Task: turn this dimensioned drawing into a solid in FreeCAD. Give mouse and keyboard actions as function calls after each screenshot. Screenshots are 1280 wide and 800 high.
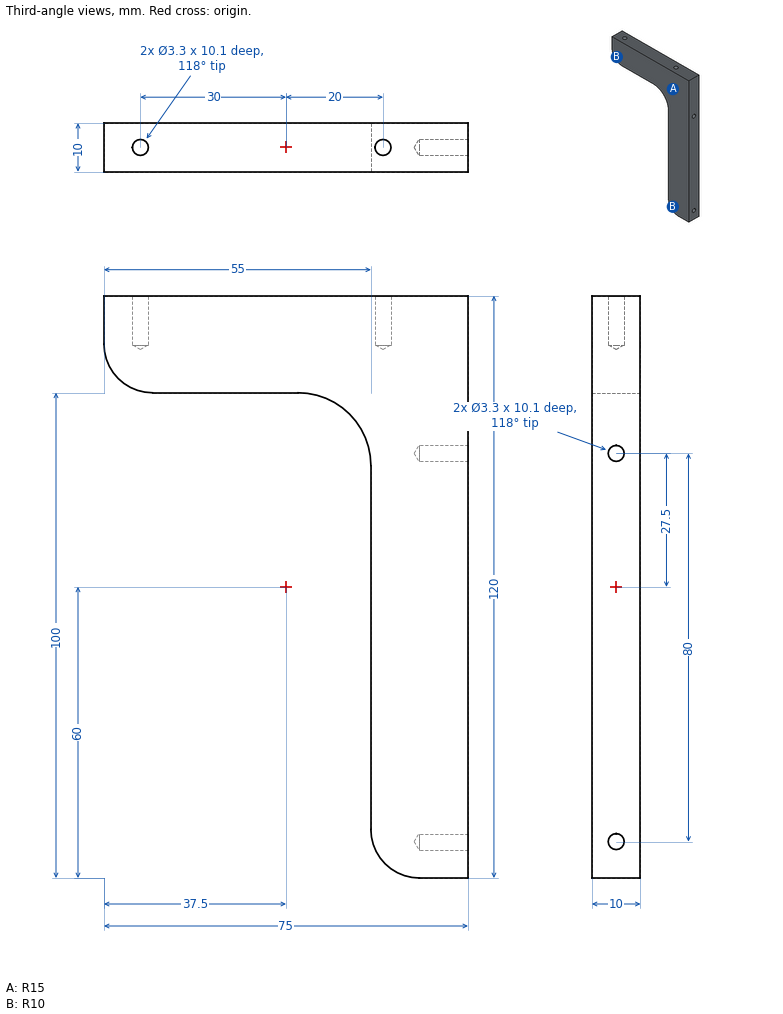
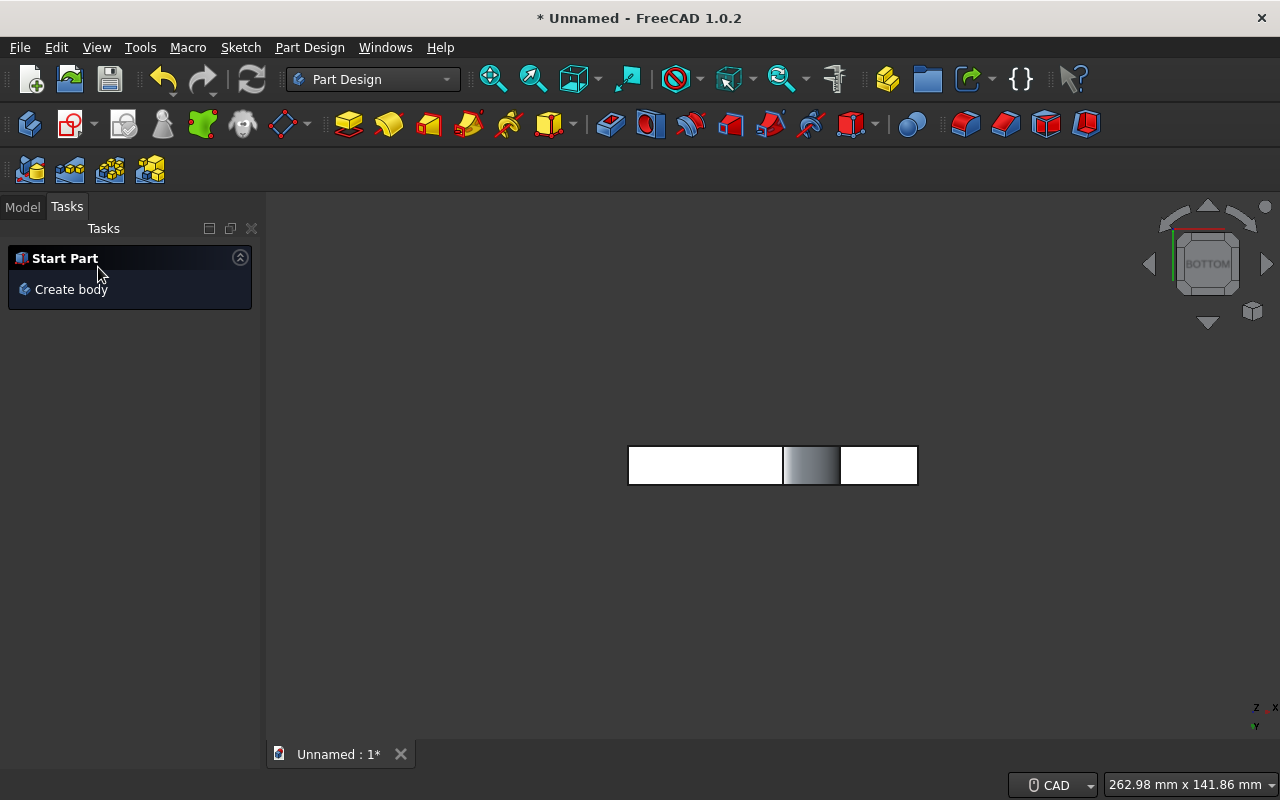
click(840, 464)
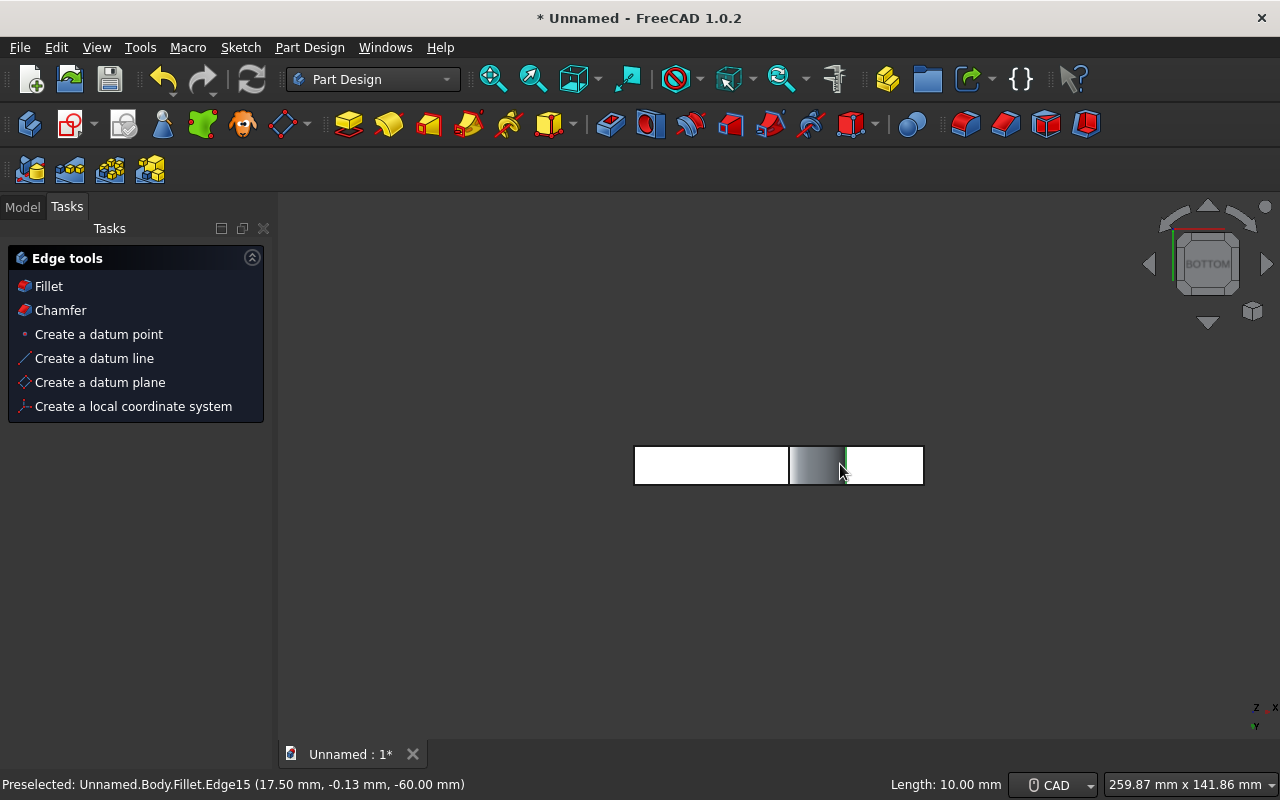
click(634, 464, ctrl)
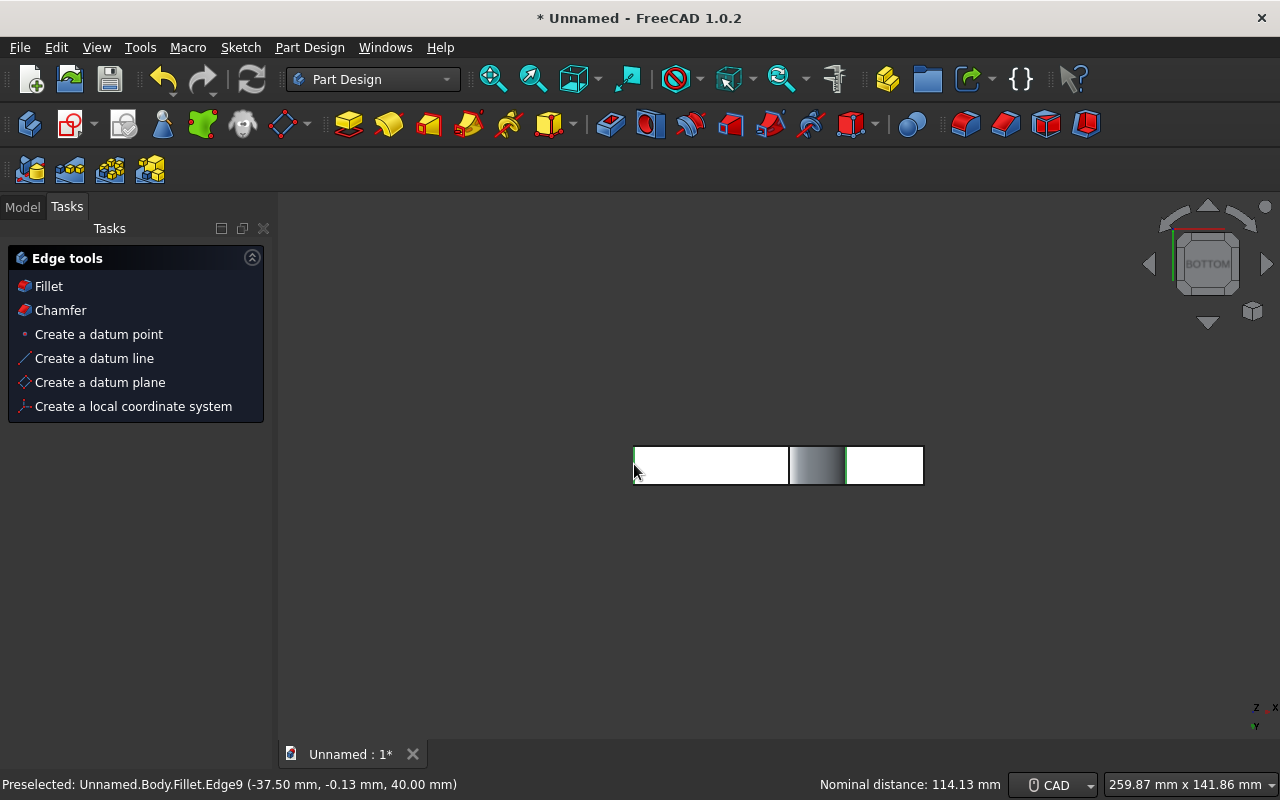
click(966, 124)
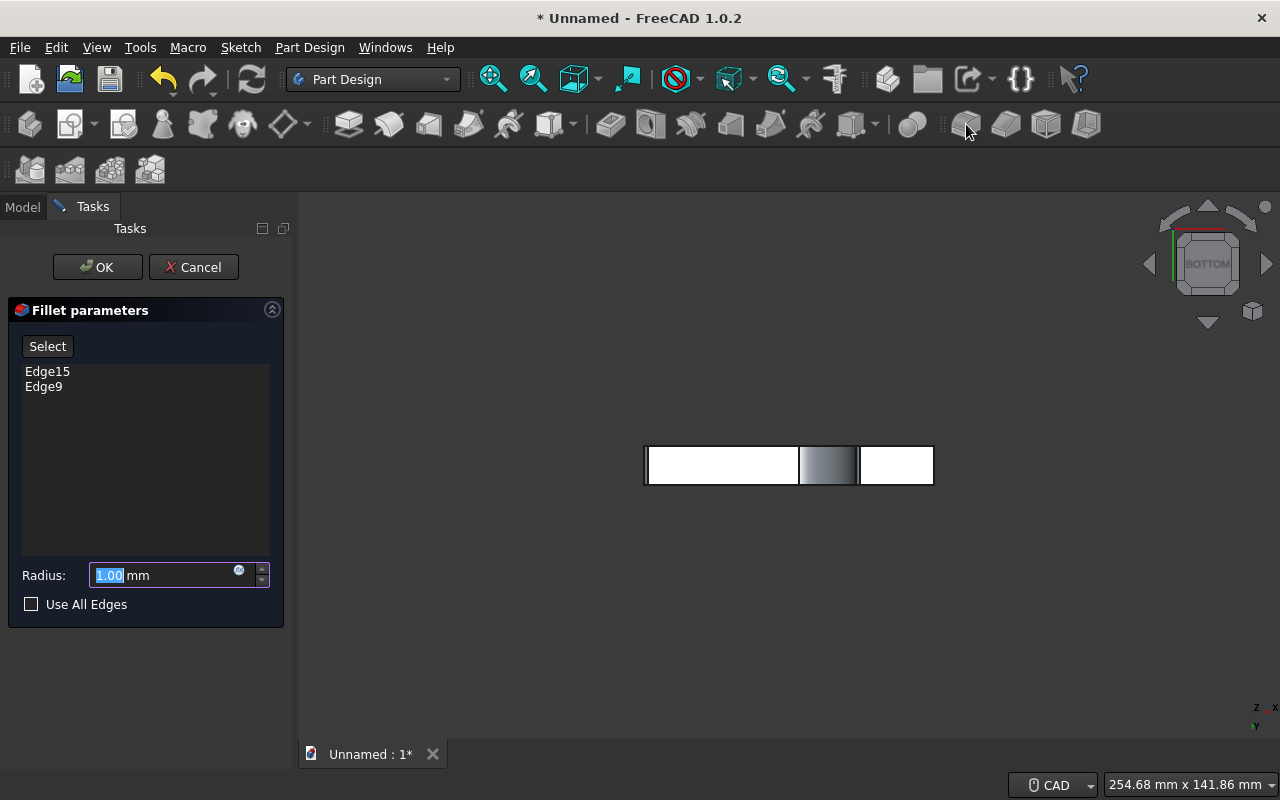
text(10)
key(Tab)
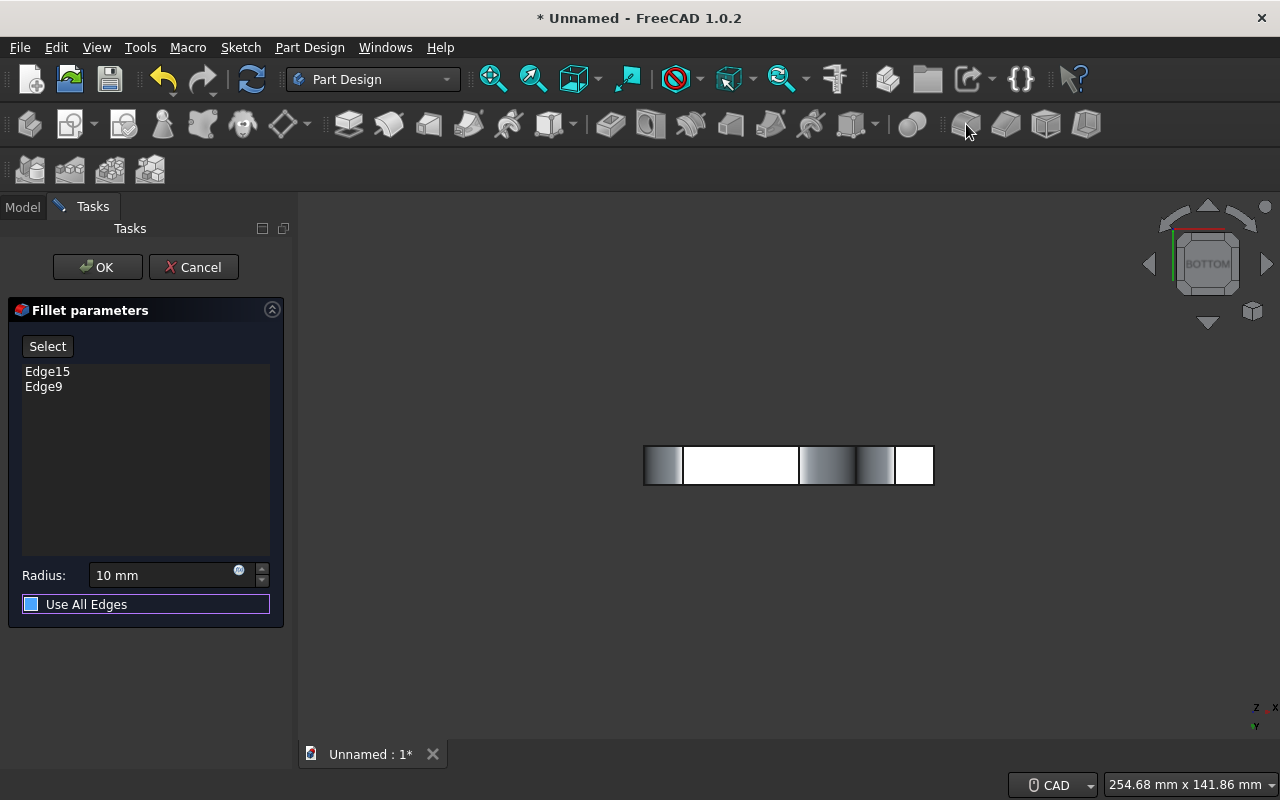
click(98, 267)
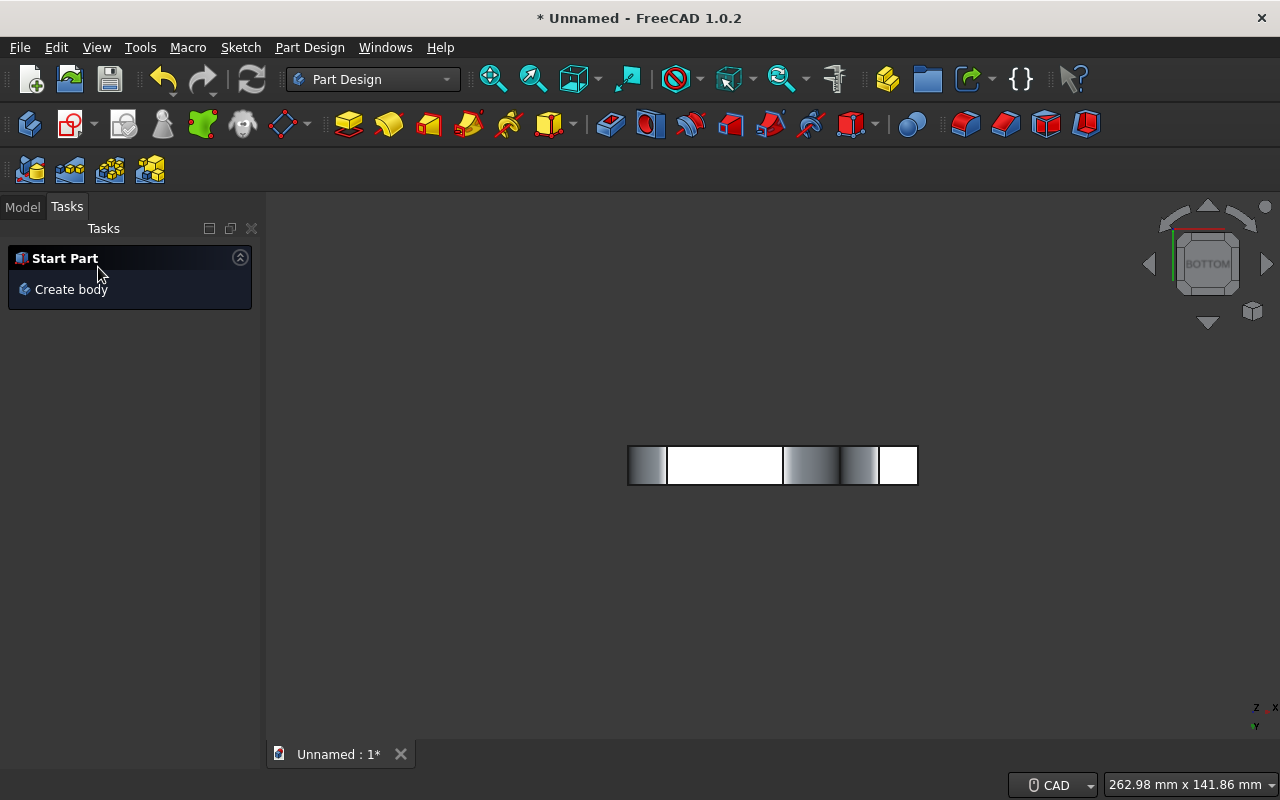
key(v)
key(f)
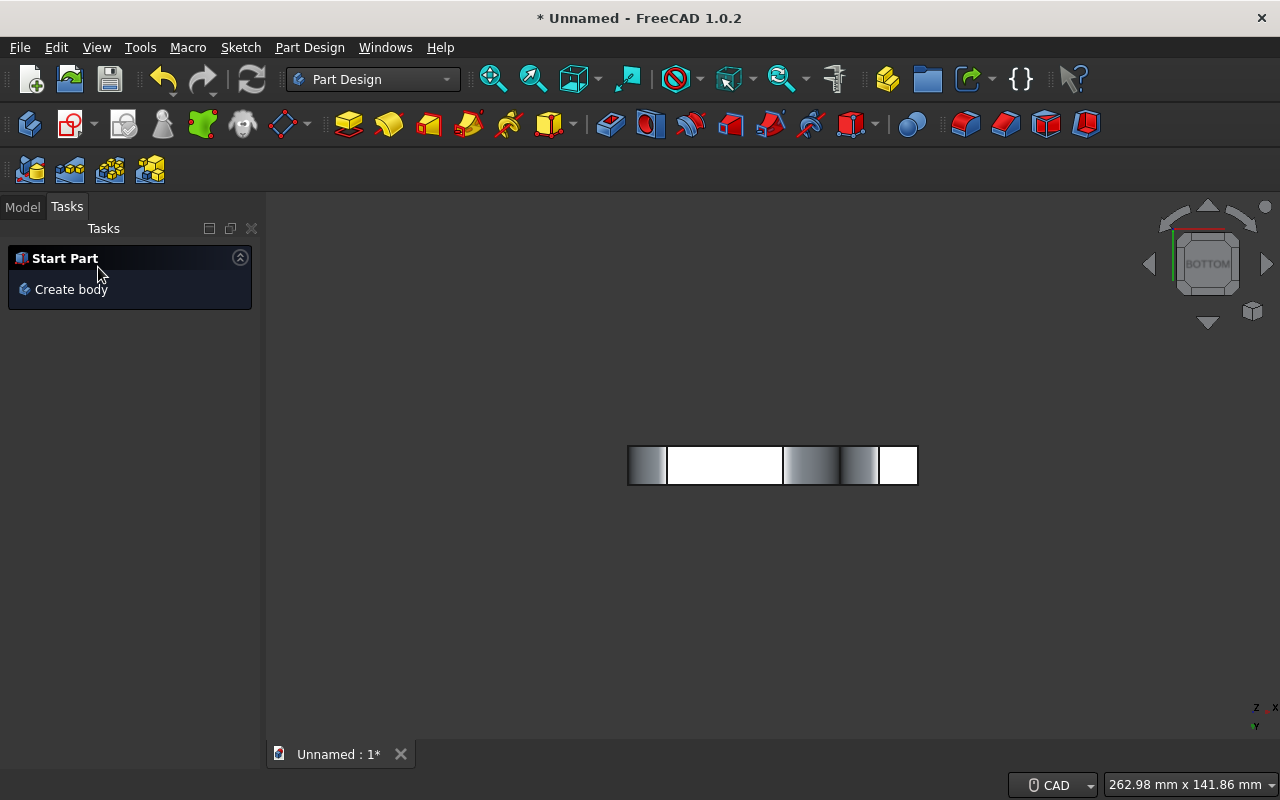
key(0)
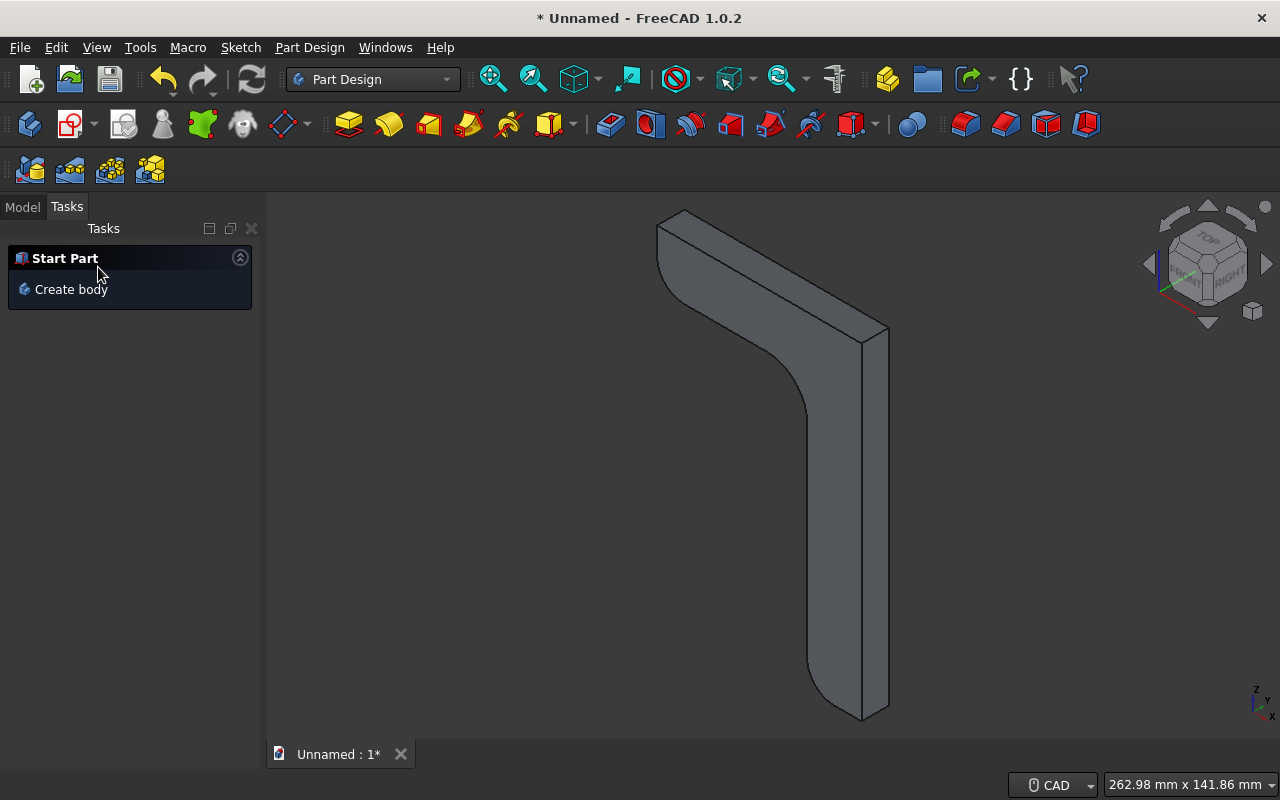
click(861, 326)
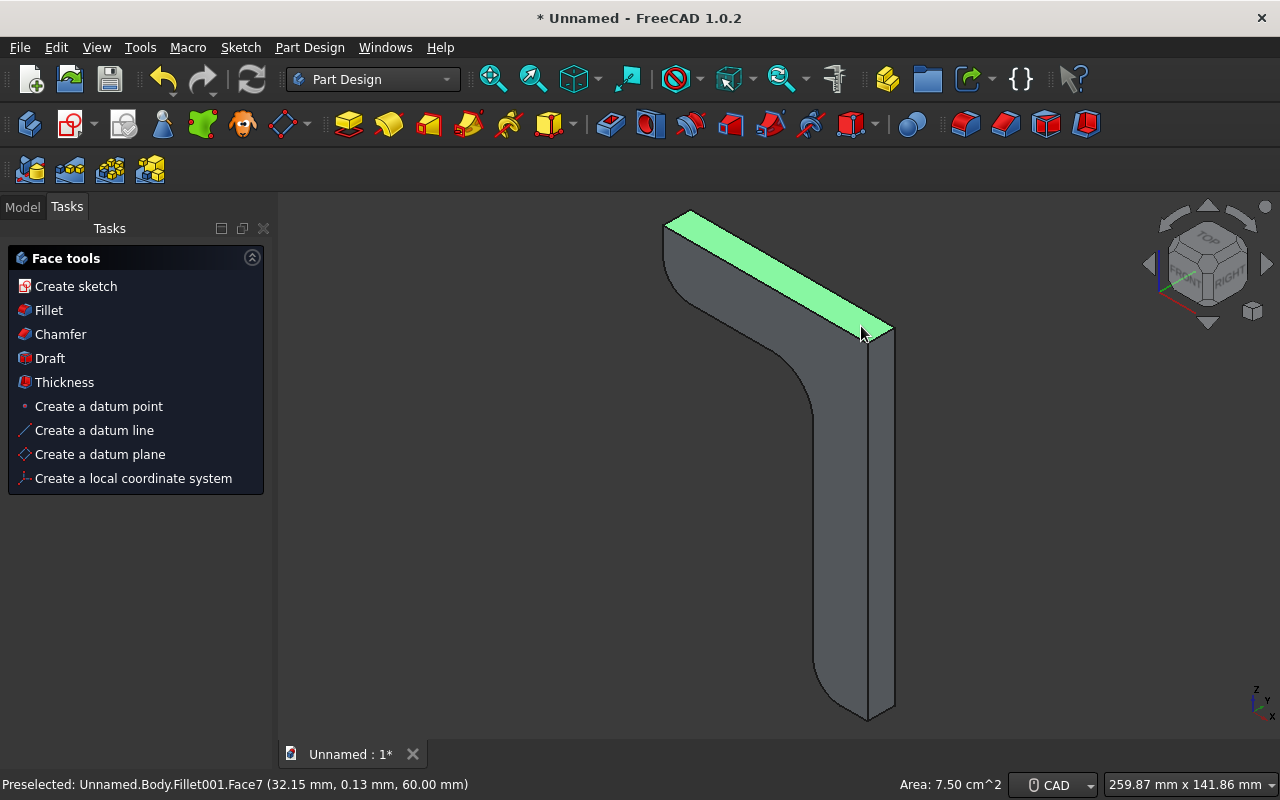
click(70, 124)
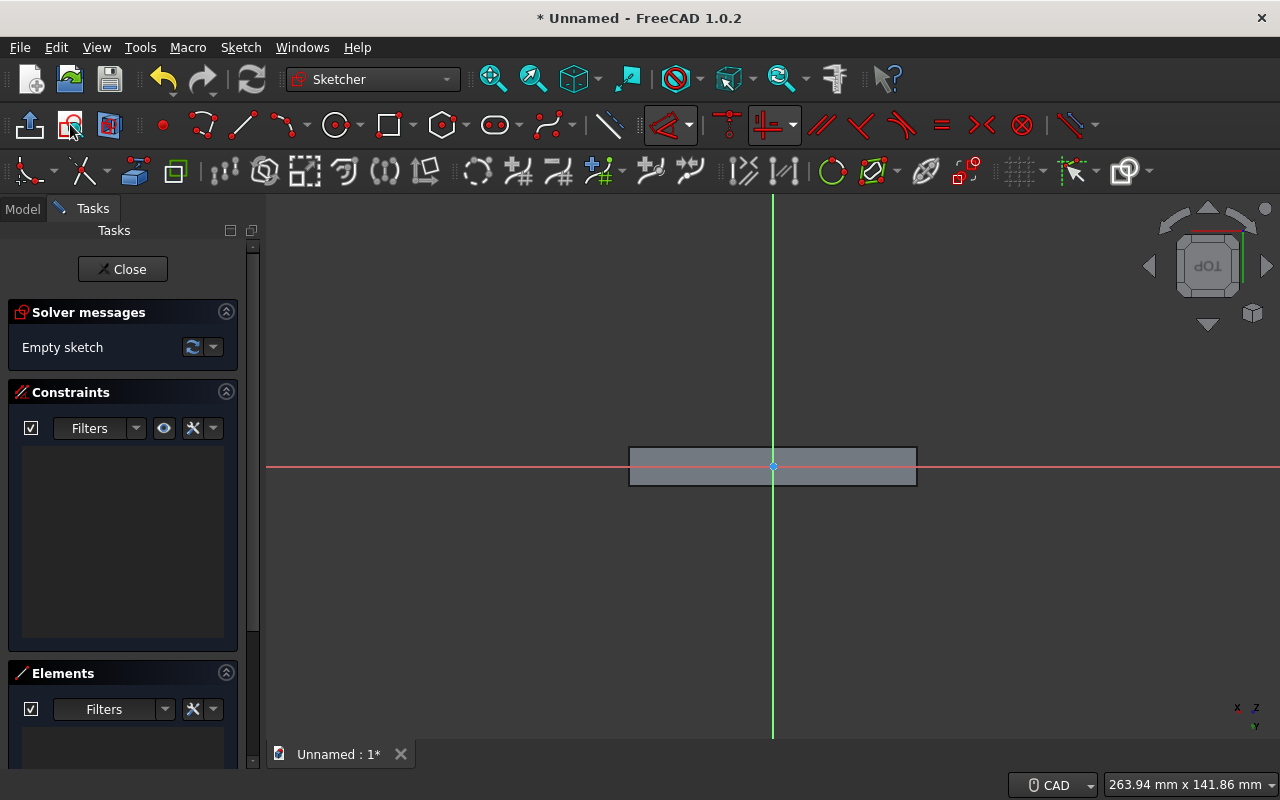
scroll(843, 467, up, 5)